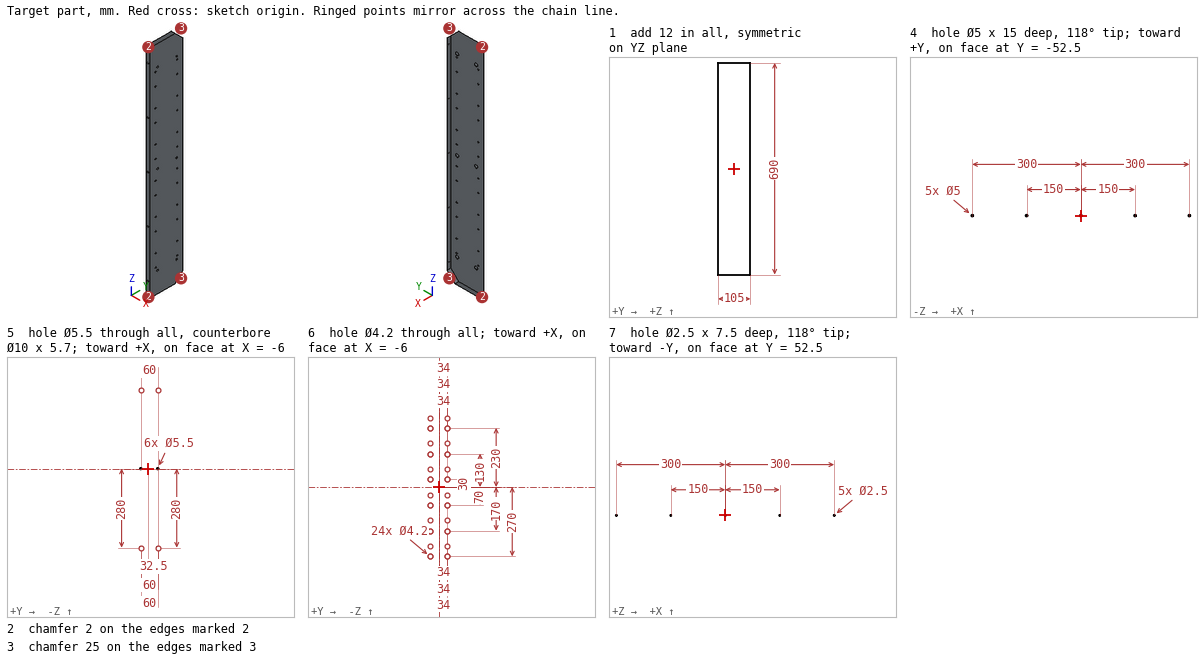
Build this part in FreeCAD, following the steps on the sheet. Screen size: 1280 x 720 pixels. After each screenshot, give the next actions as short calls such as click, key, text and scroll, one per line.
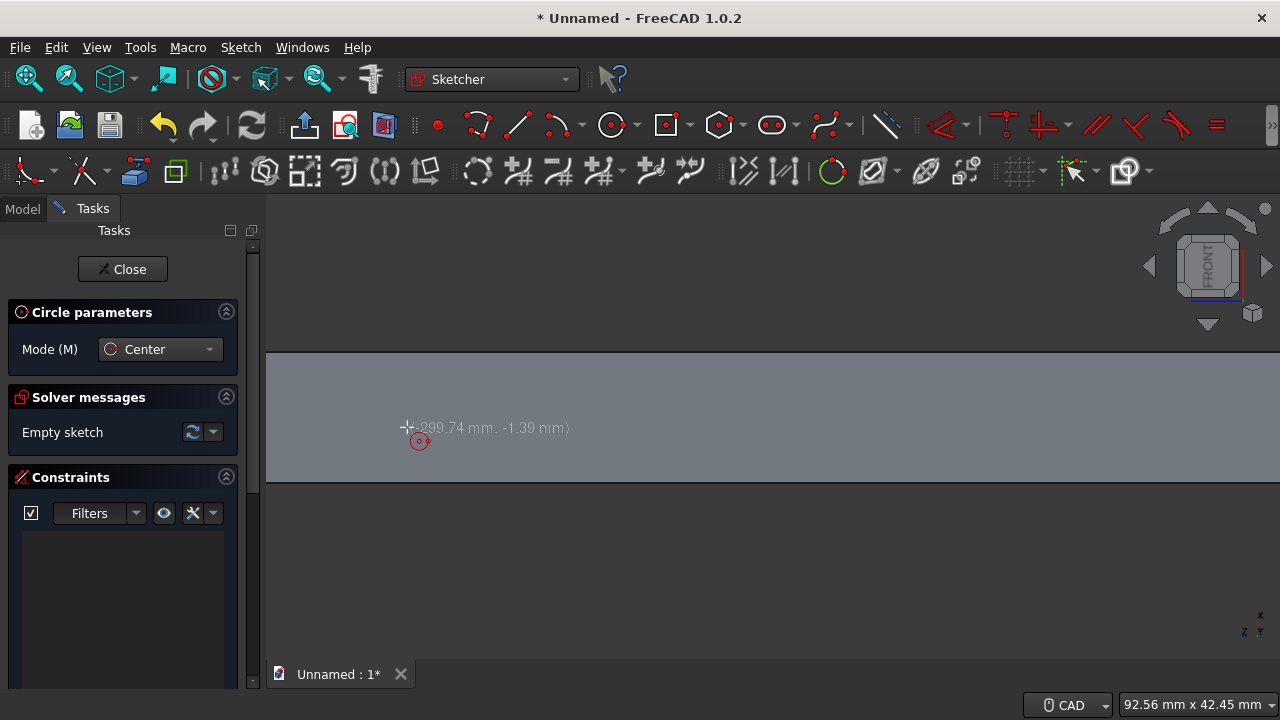
scroll(407, 427, down, 12)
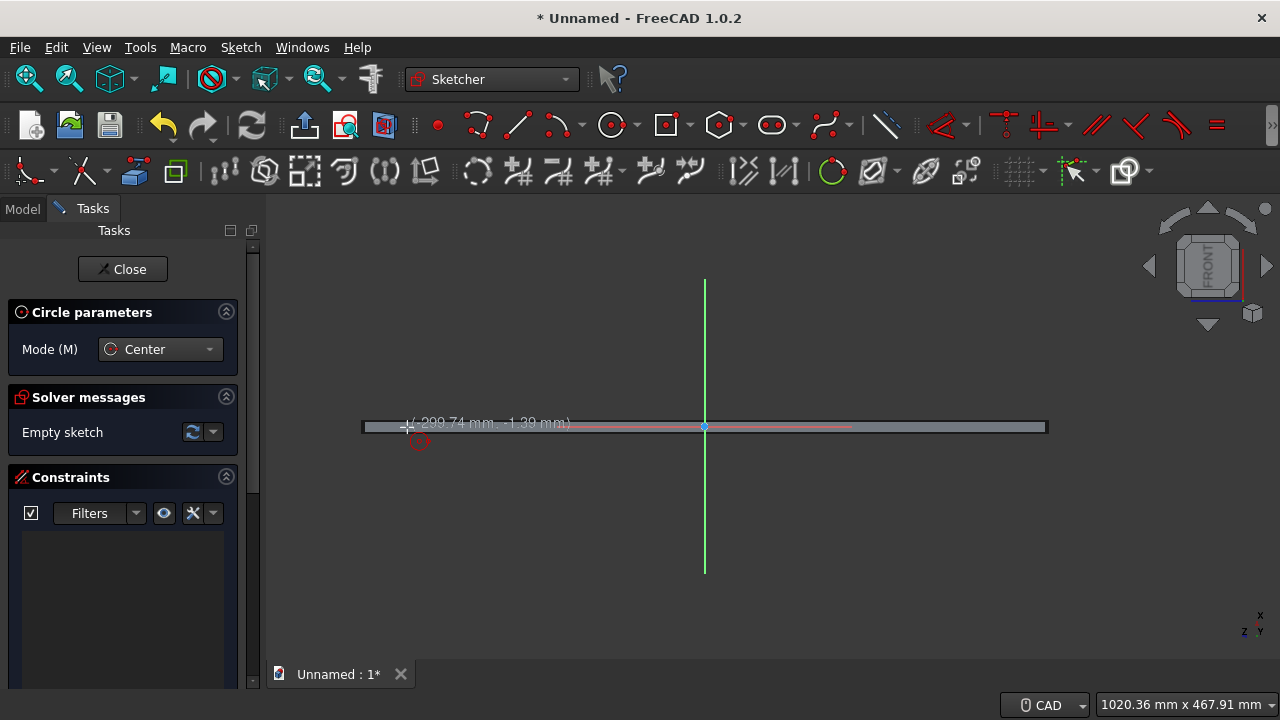
click(407, 427)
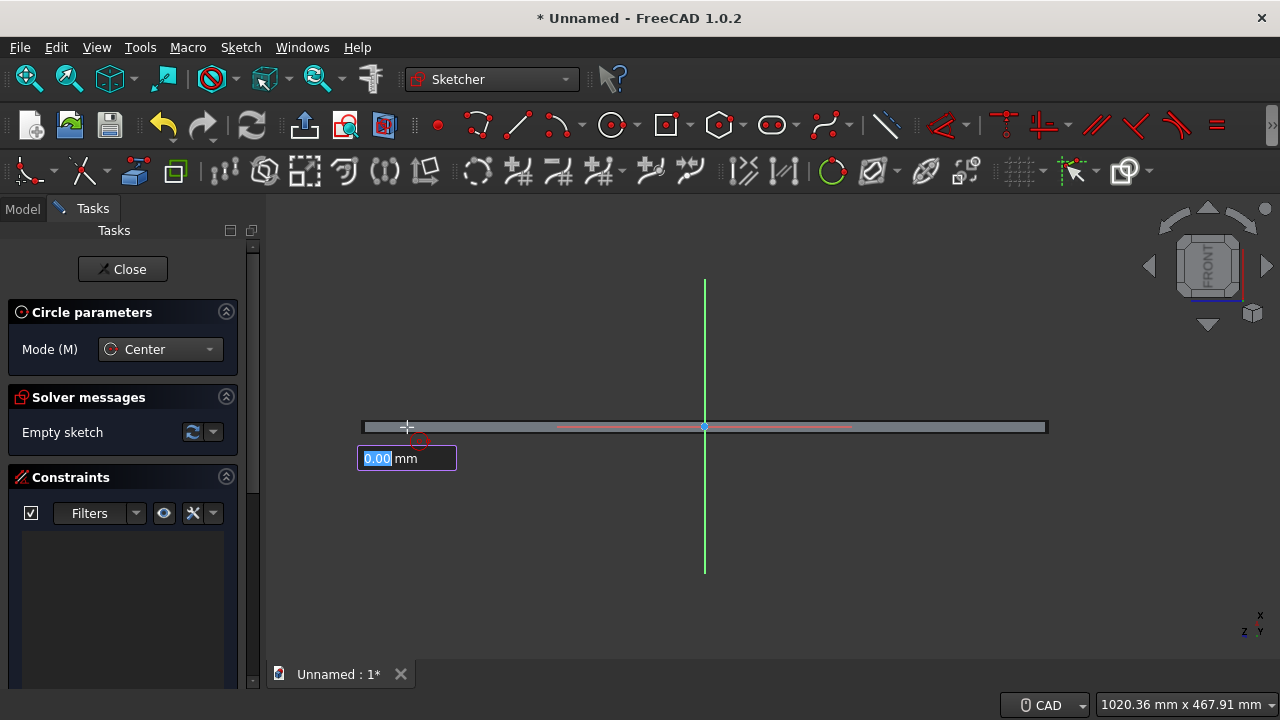
scroll(406, 429, up, 10)
move(404, 425)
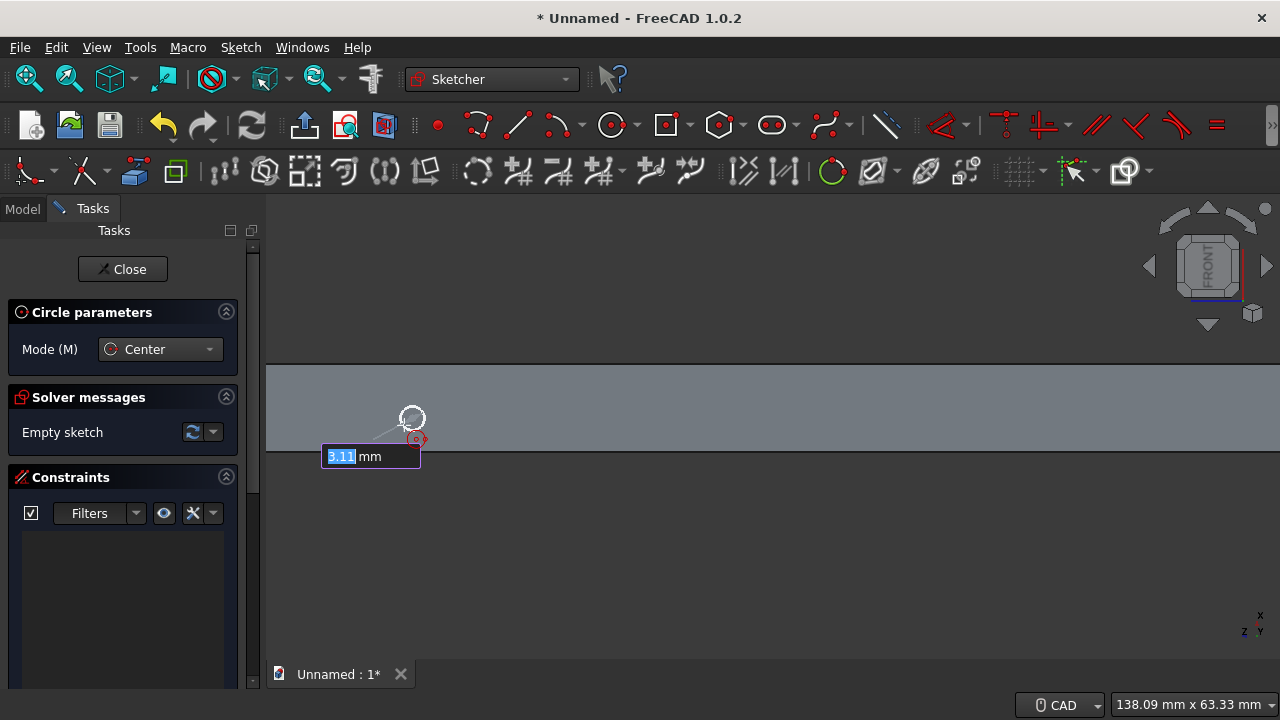
text(5)
key(Return)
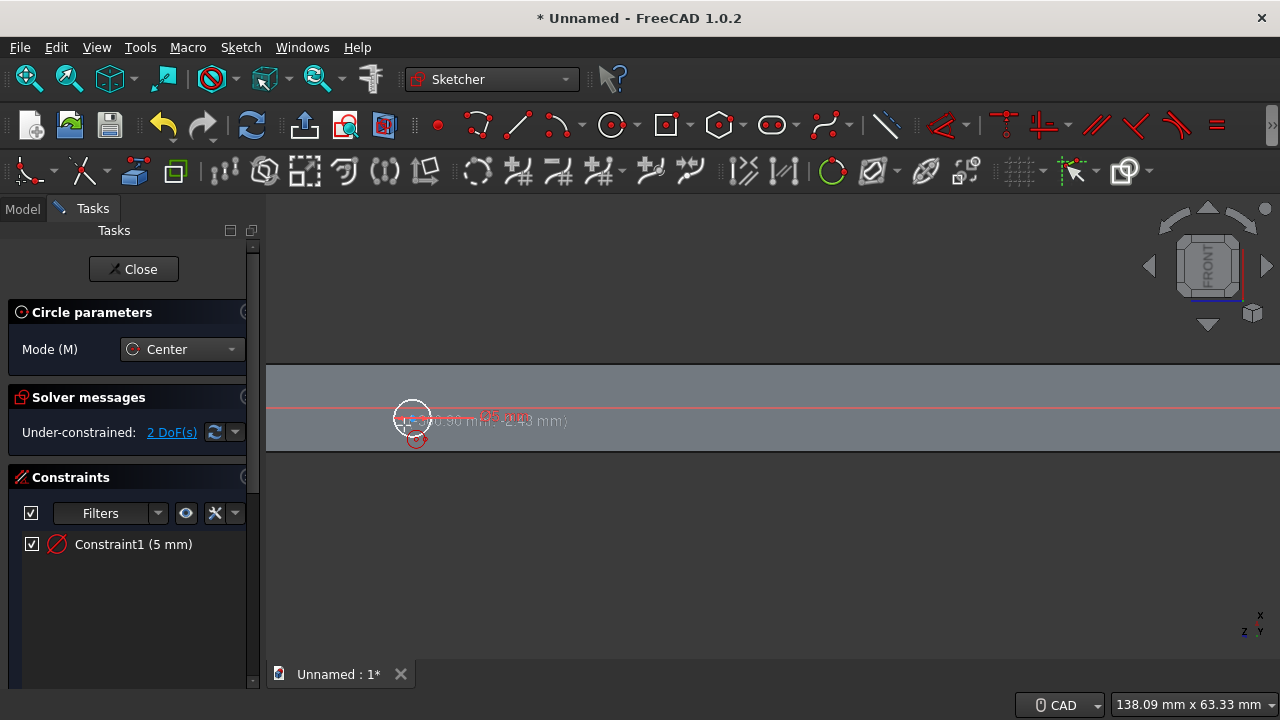
scroll(406, 429, down, 10)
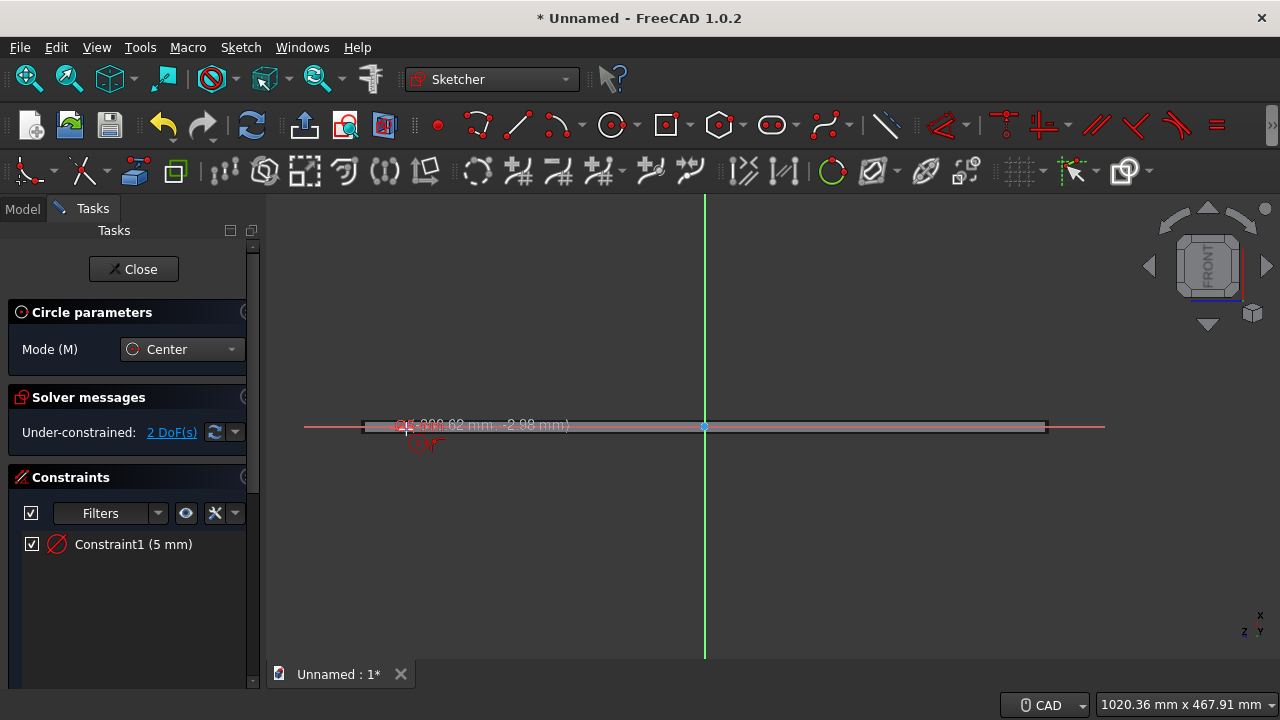
scroll(556, 427, up, 12)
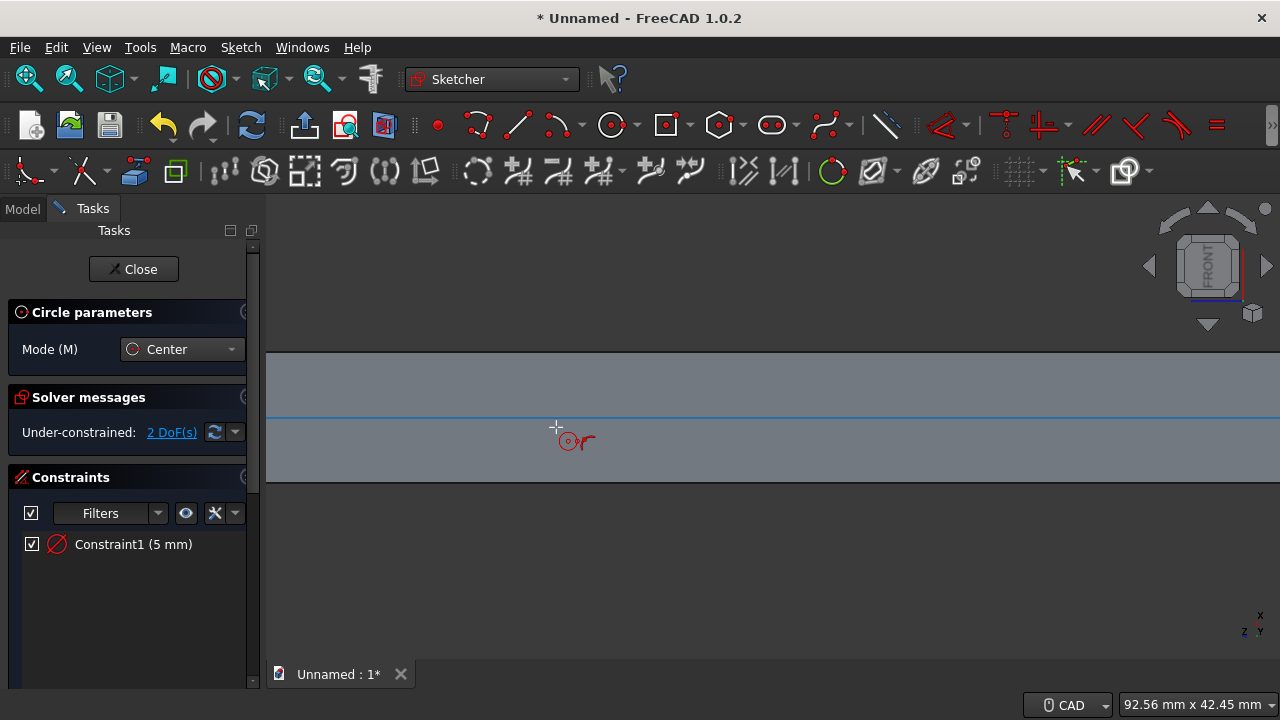
scroll(556, 427, down, 12)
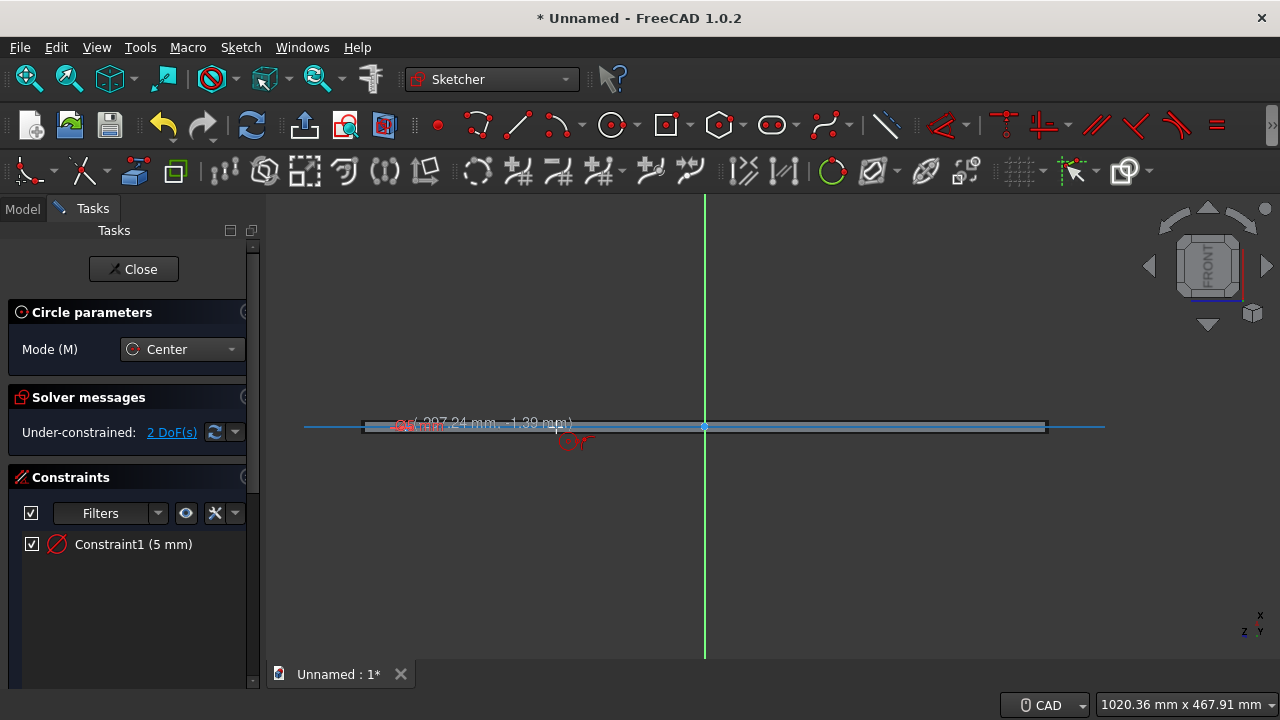
click(556, 427)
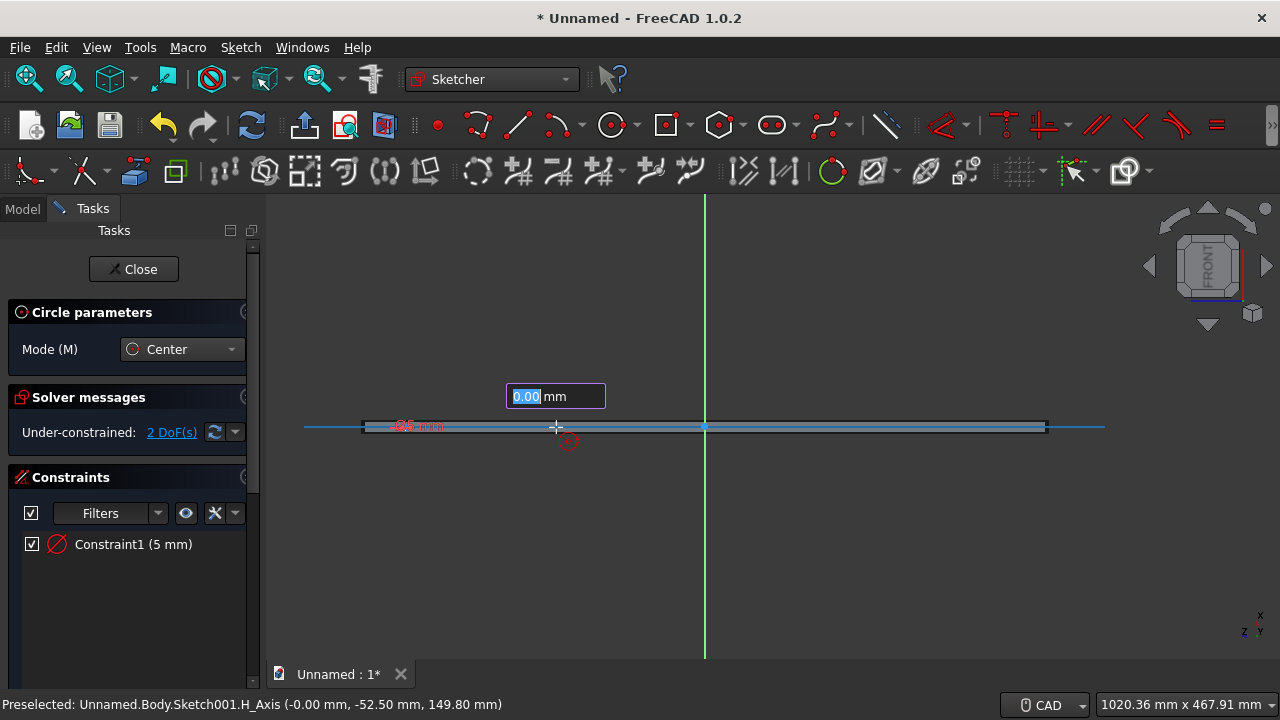
scroll(555, 429, up, 10)
move(553, 425)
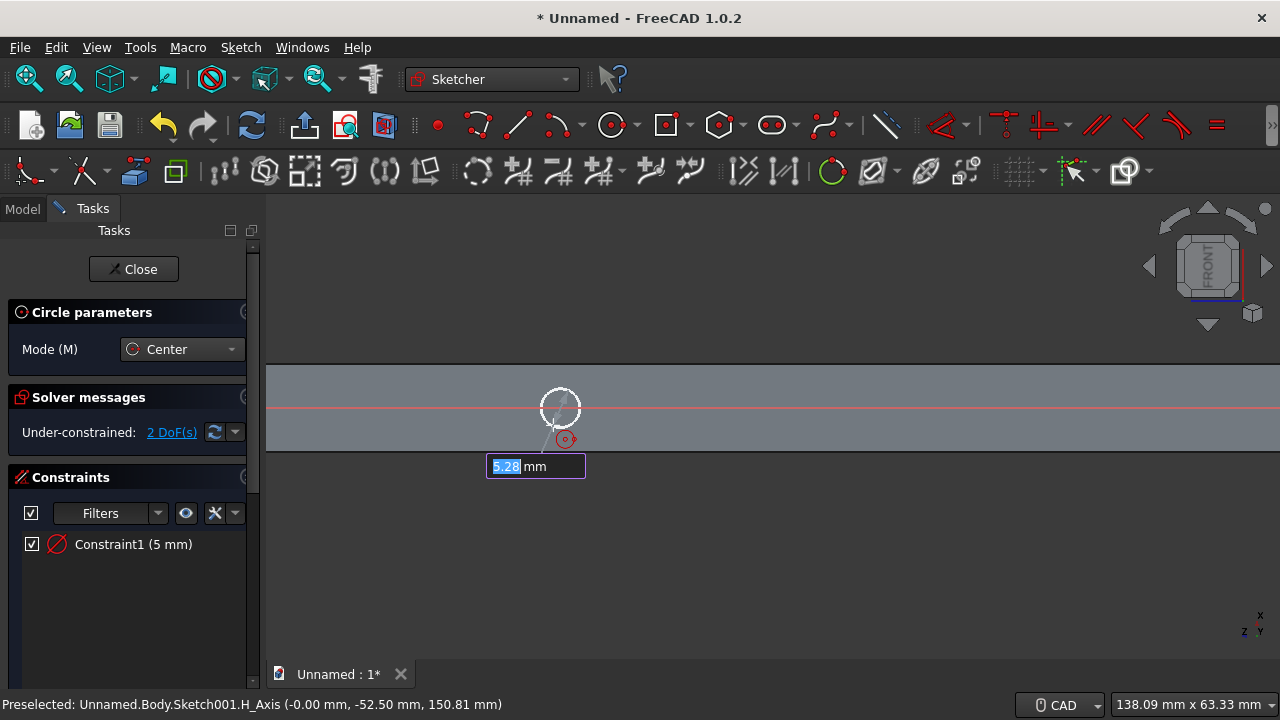
text(5)
key(Return)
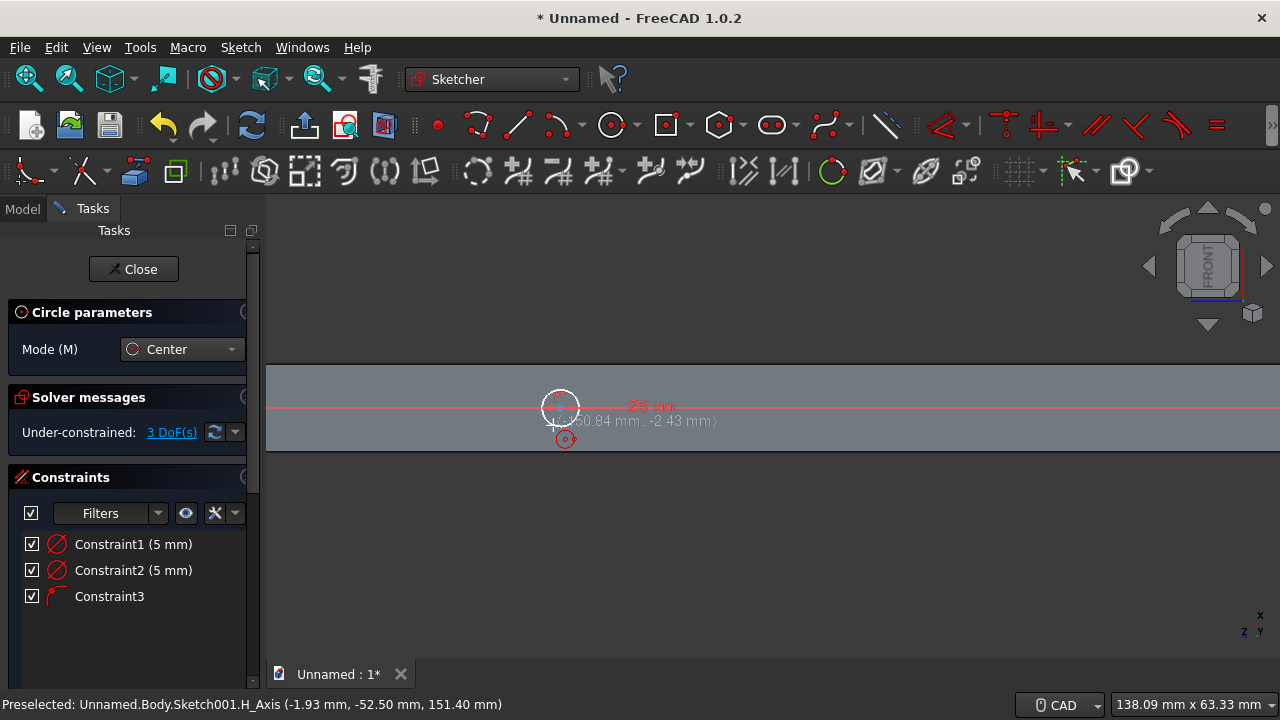
scroll(555, 429, down, 10)